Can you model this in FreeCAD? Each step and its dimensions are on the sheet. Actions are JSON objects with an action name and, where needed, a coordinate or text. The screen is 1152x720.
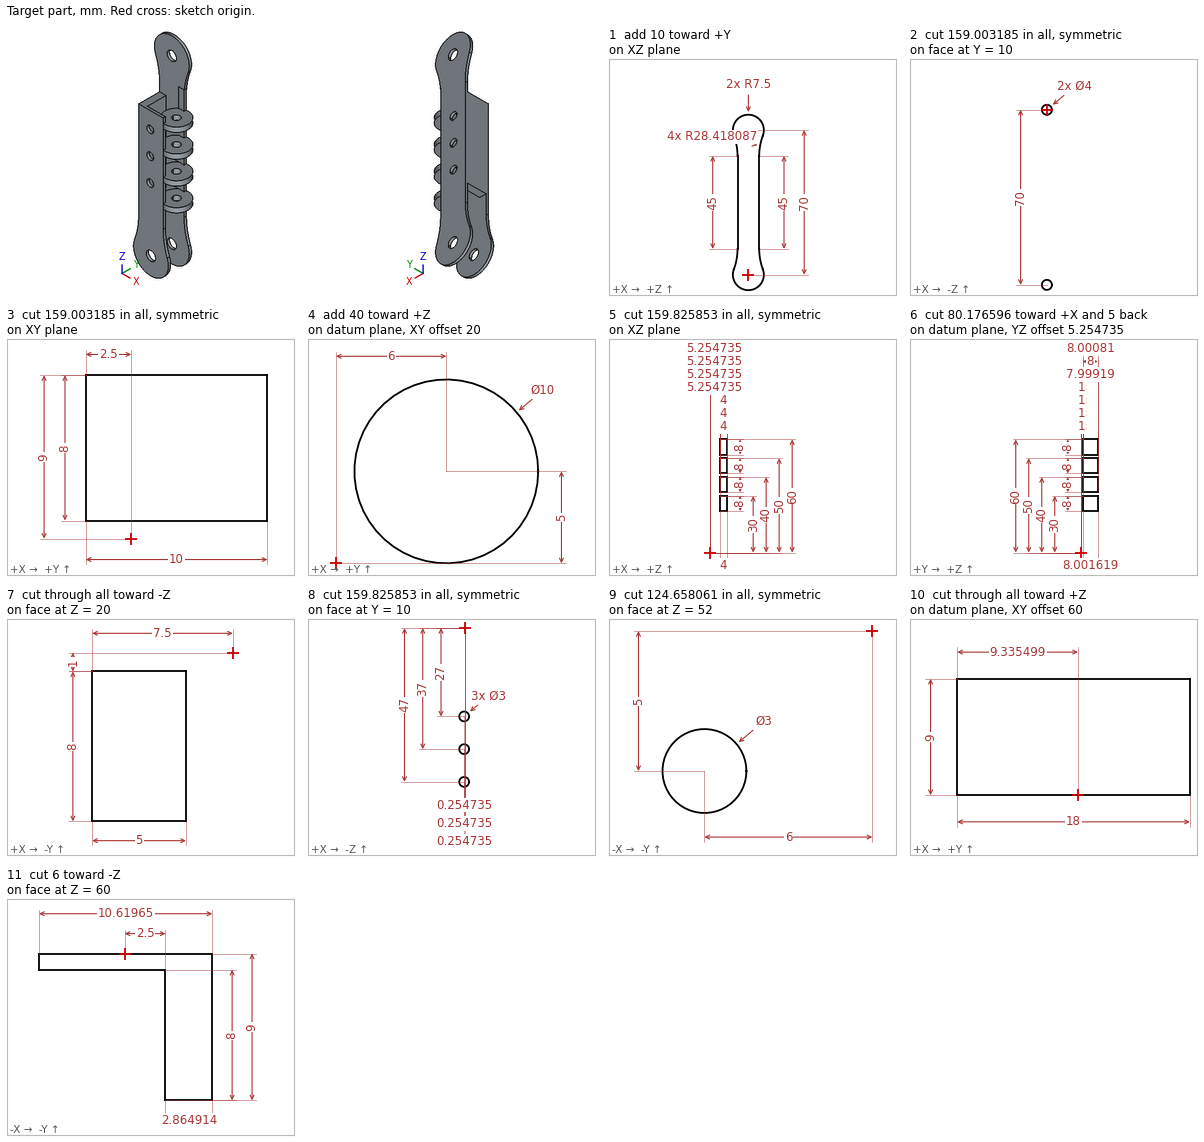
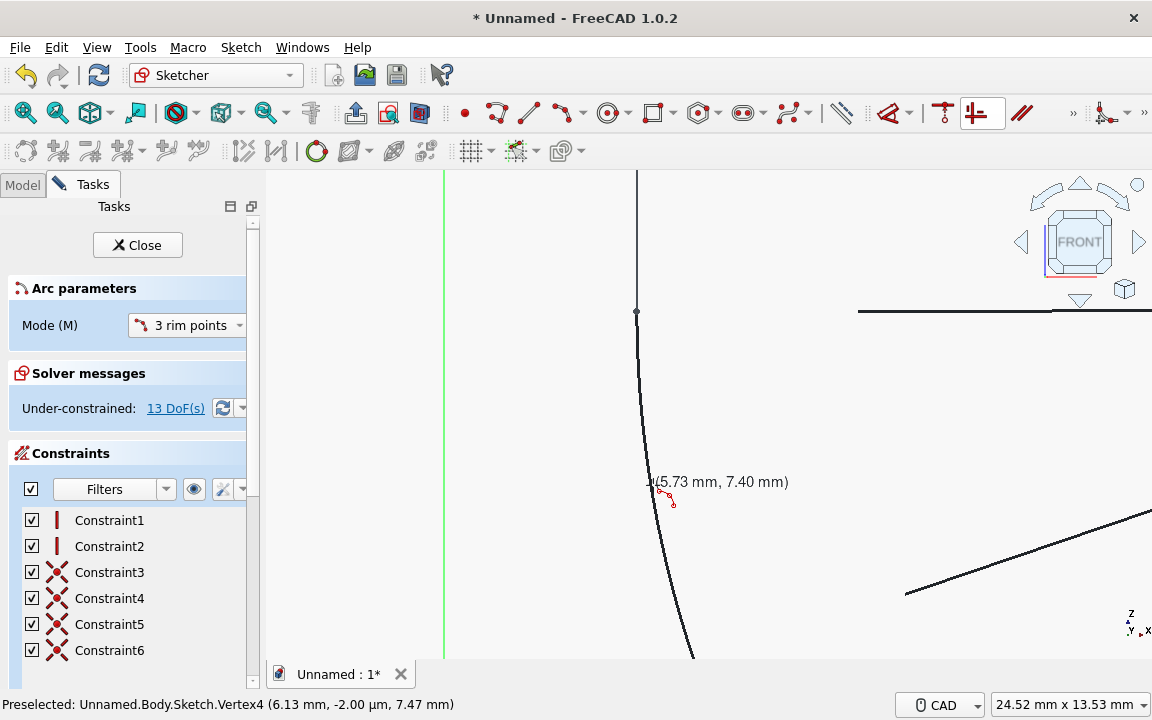
{"action": "left_click", "coordinate": [650, 485]}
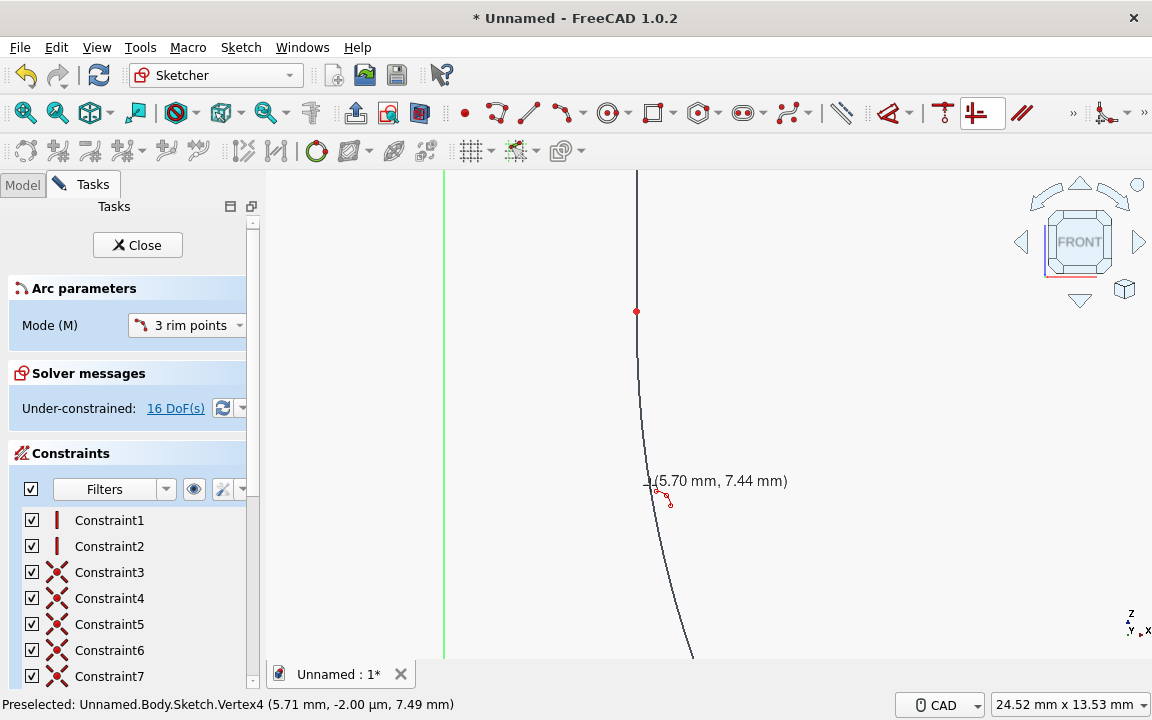
{"action": "scroll", "coordinate": [660, 507], "scroll_direction": "down", "scroll_amount": 12}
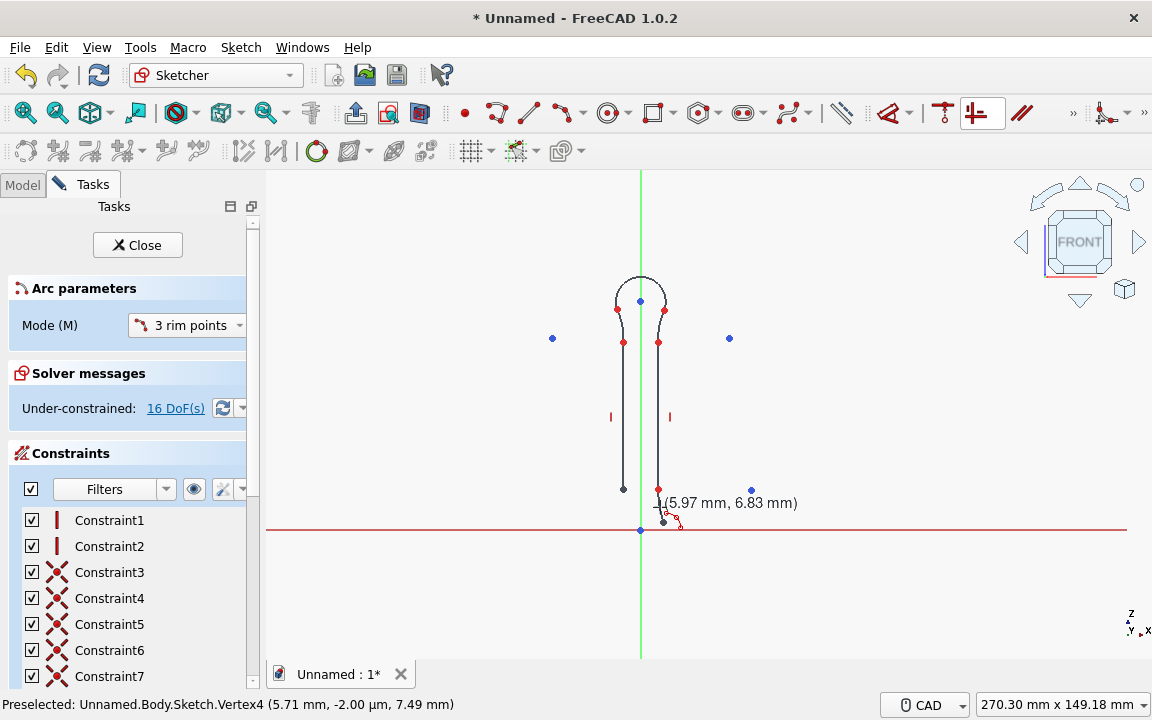
{"action": "scroll", "coordinate": [664, 522], "scroll_direction": "up", "scroll_amount": 4}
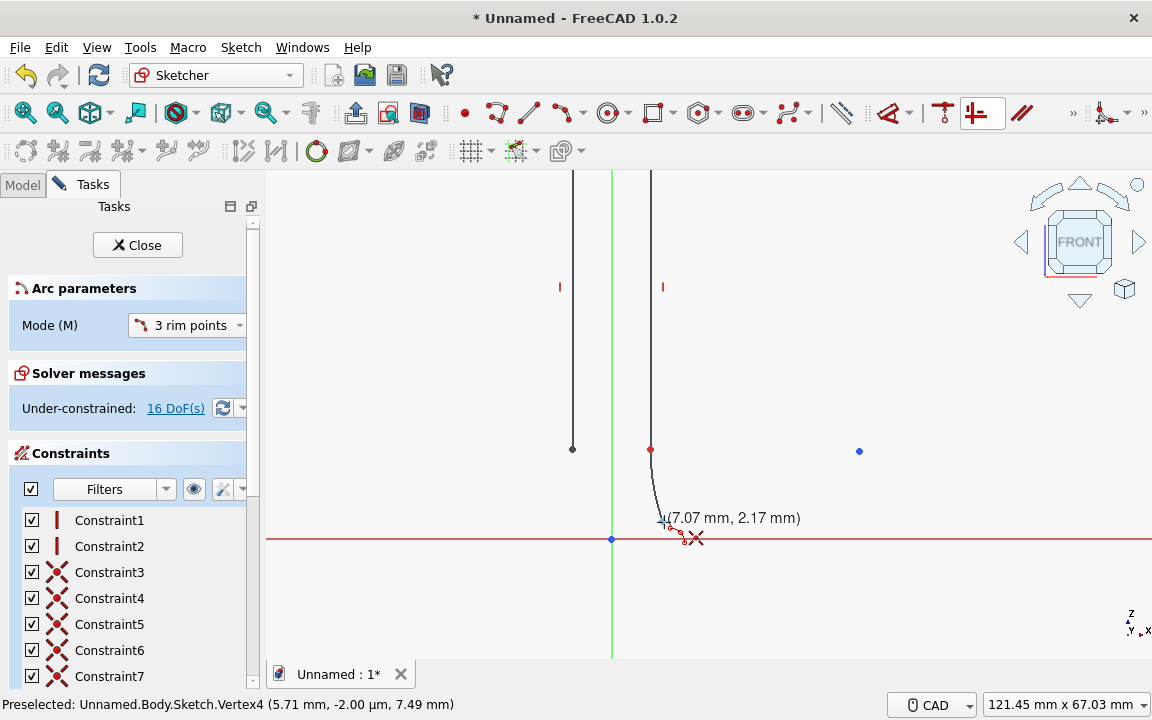
{"action": "left_click", "coordinate": [663, 521]}
{"action": "left_click", "coordinate": [561, 520]}
{"action": "left_click", "coordinate": [574, 578]}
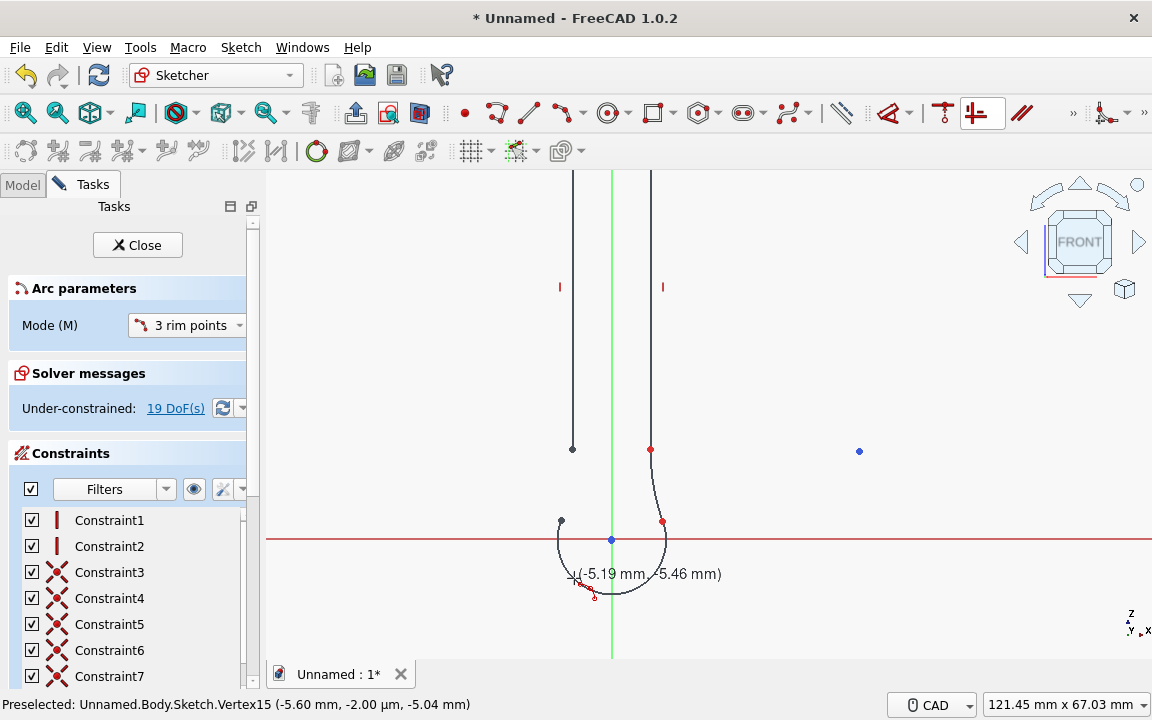
{"action": "left_click", "coordinate": [561, 521]}
{"action": "left_click", "coordinate": [573, 450]}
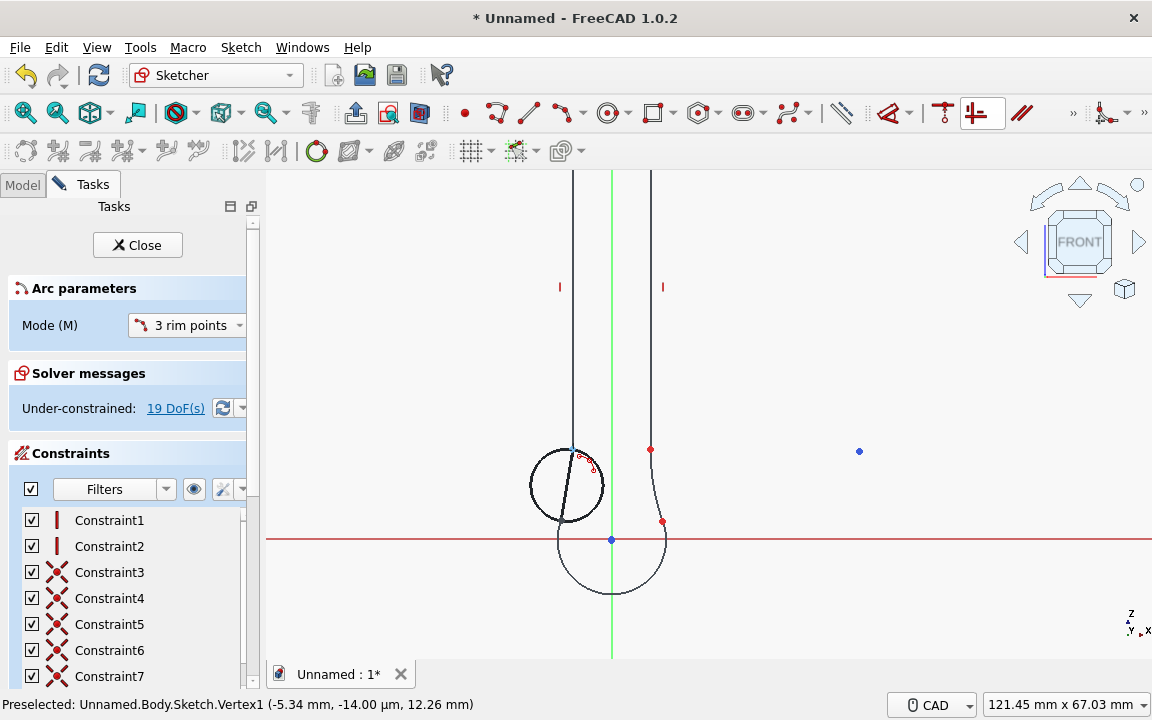
{"action": "scroll", "coordinate": [570, 485], "scroll_direction": "up", "scroll_amount": 8}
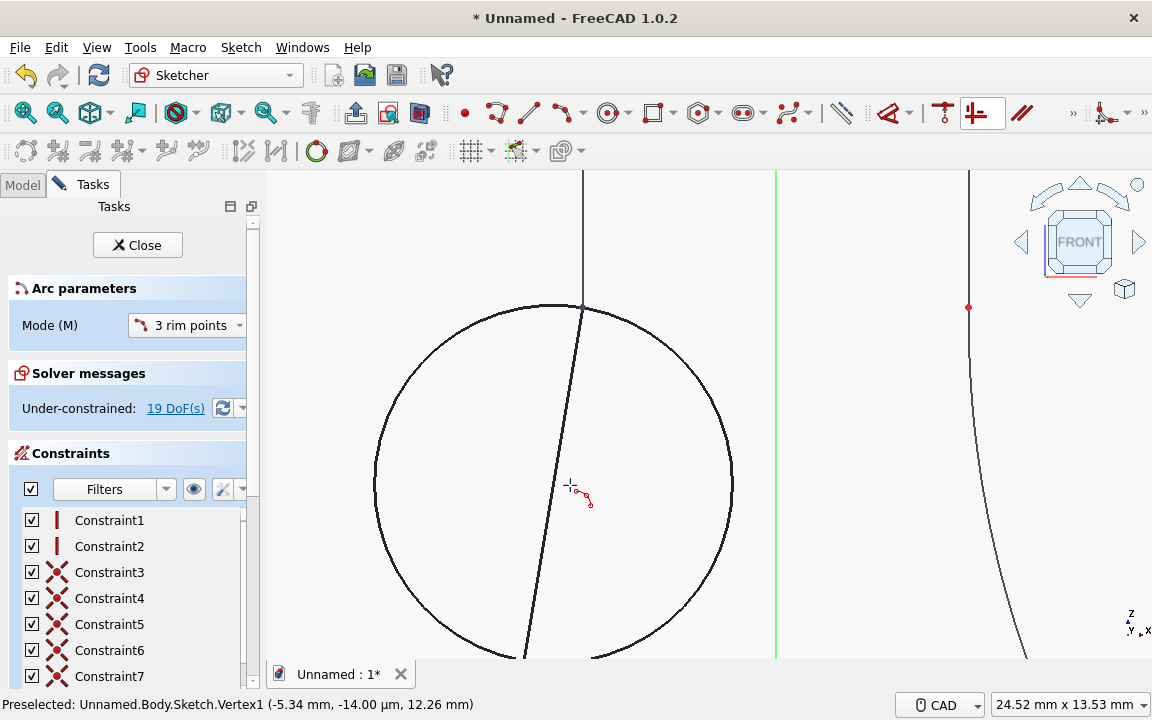
{"action": "left_click", "coordinate": [570, 481]}
{"action": "key", "text": "Escape"}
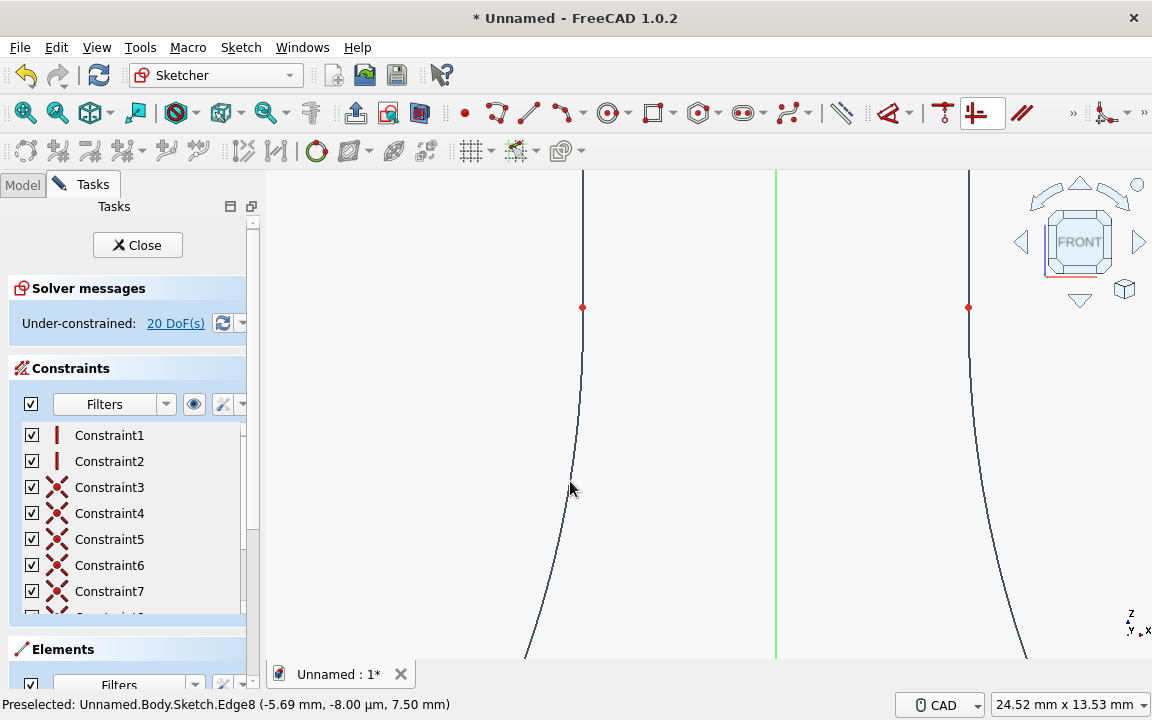
{"action": "scroll", "coordinate": [627, 507], "scroll_direction": "down", "scroll_amount": 12}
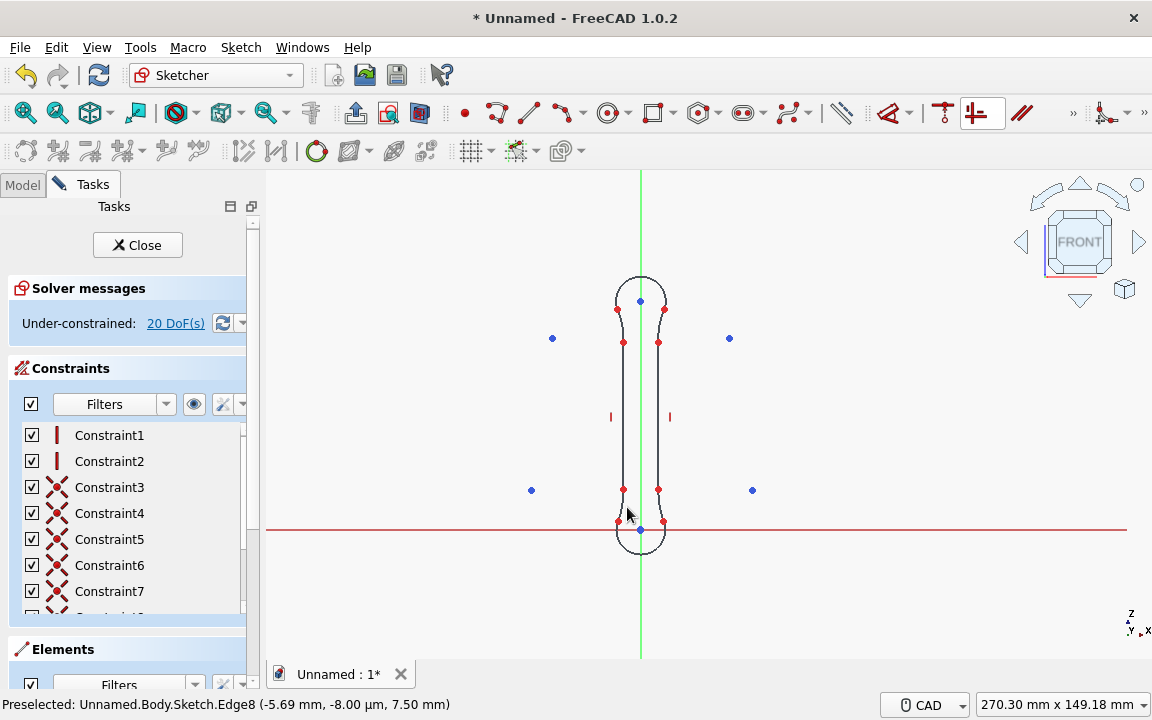
{"action": "left_click", "coordinate": [623, 445]}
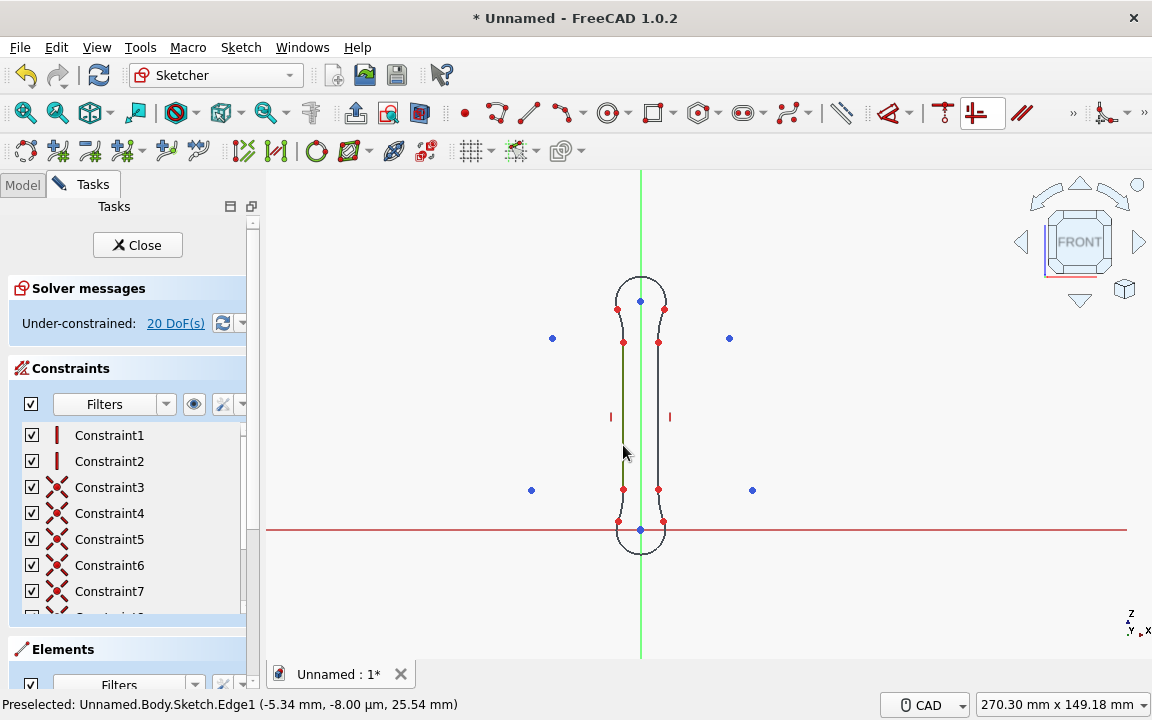
{"action": "scroll", "coordinate": [623, 332], "scroll_direction": "up", "scroll_amount": 2}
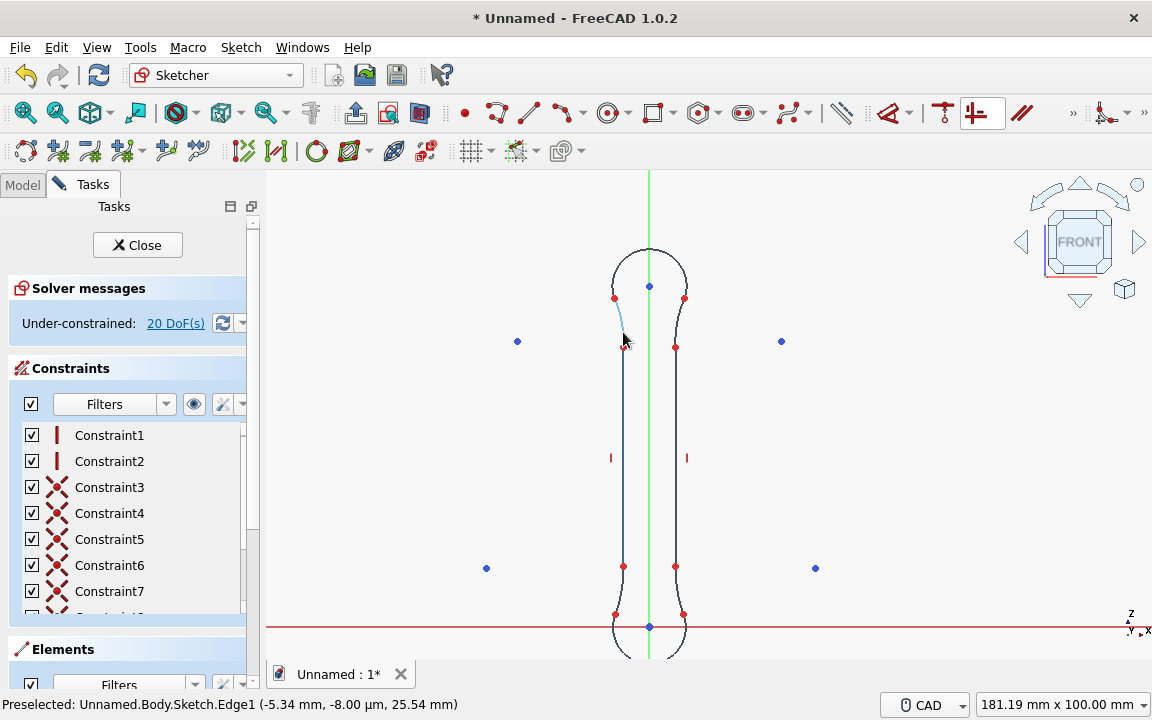
{"action": "left_click", "coordinate": [623, 332]}